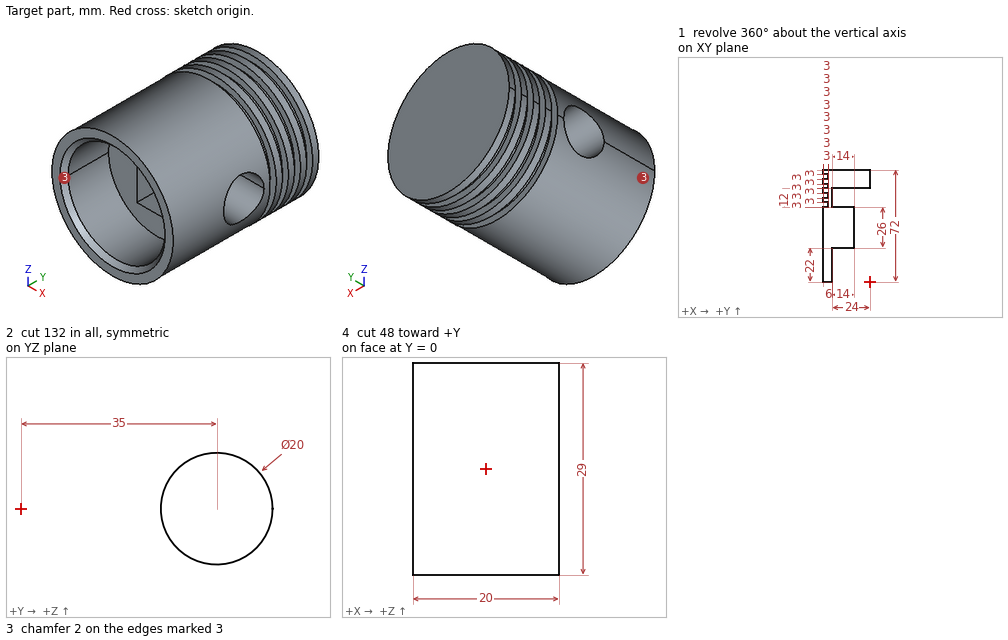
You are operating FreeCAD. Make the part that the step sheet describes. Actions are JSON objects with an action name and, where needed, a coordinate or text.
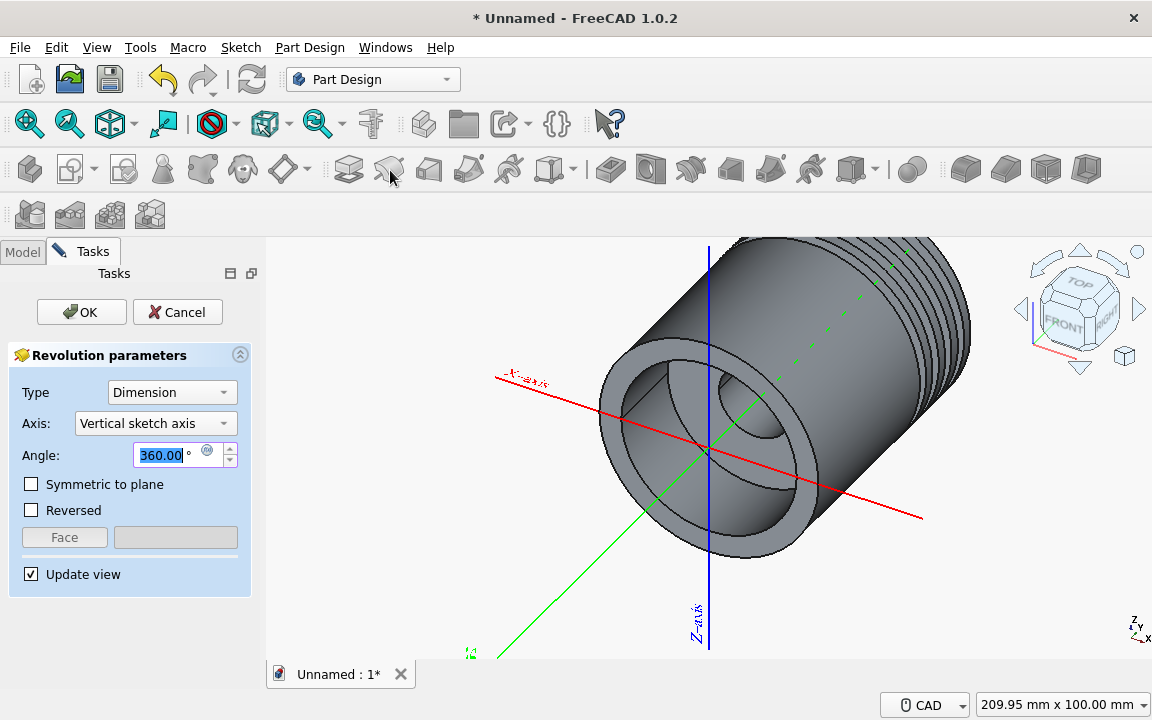
{"action": "left_click", "coordinate": [82, 312]}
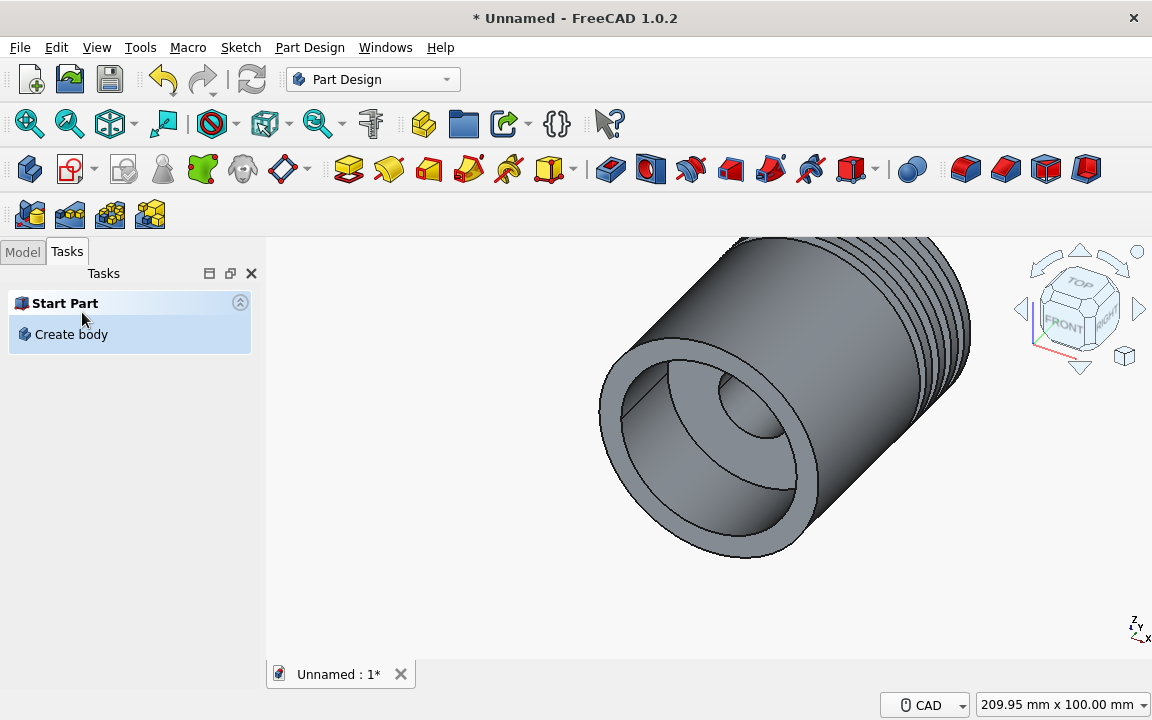
{"action": "left_click", "coordinate": [30, 124]}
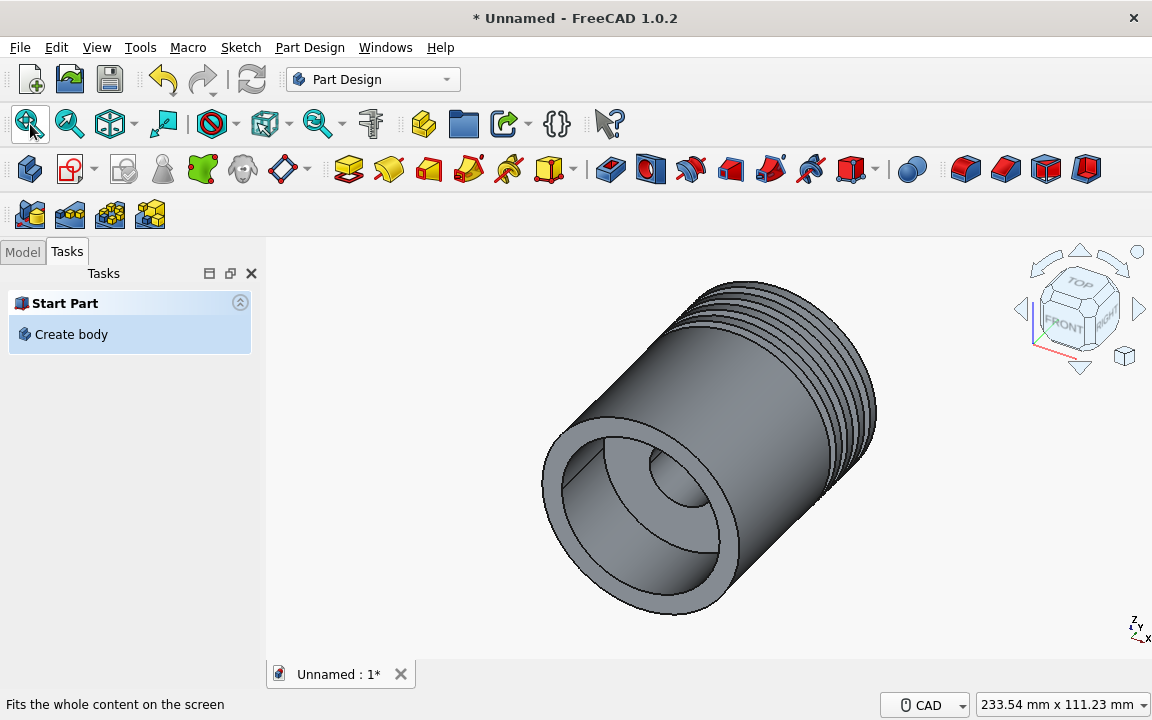
{"action": "left_click", "coordinate": [70, 170]}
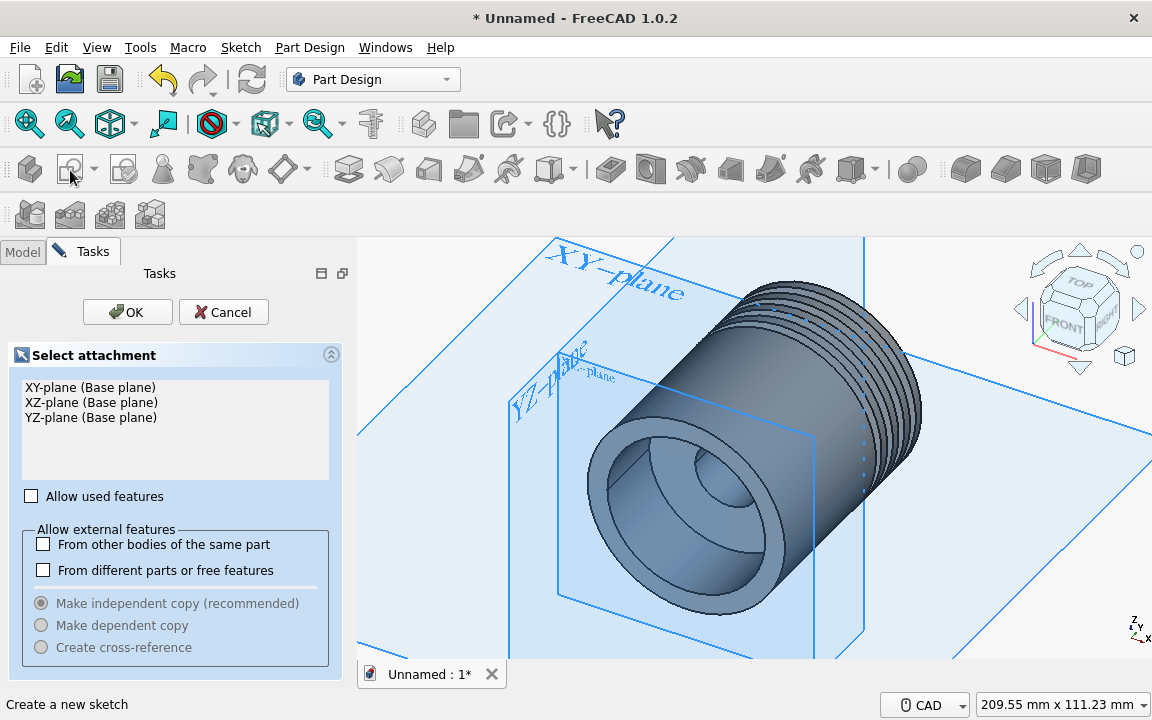
{"action": "left_click", "coordinate": [82, 418]}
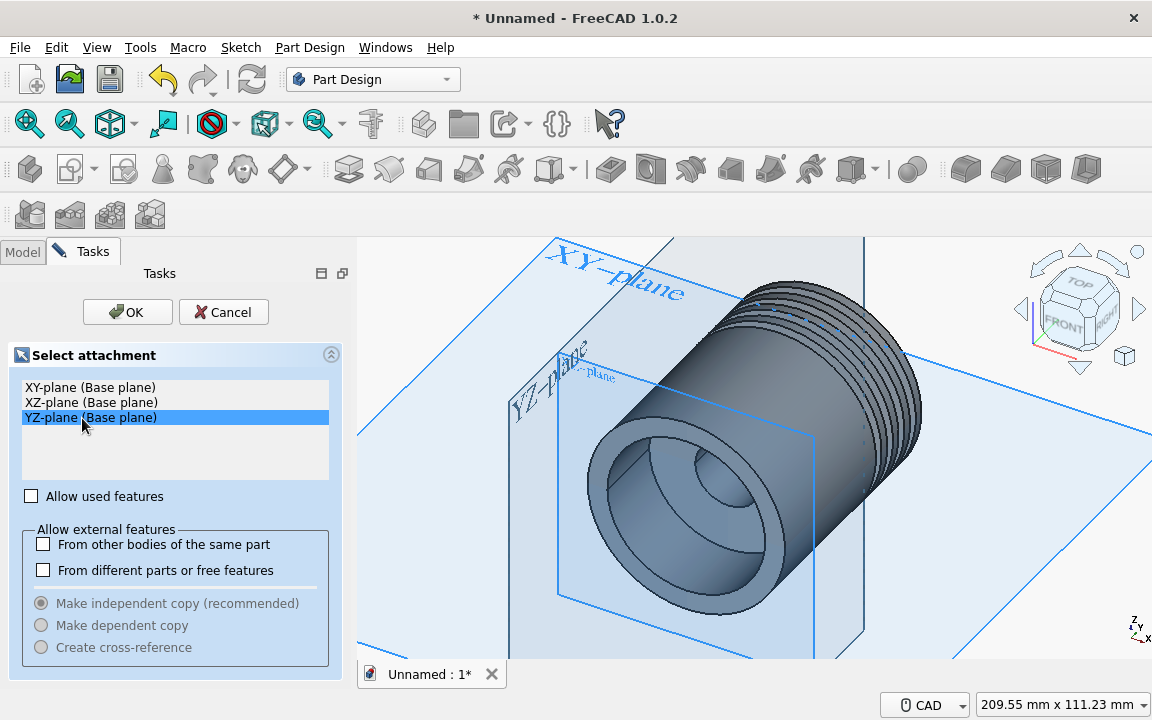
{"action": "left_click", "coordinate": [128, 312]}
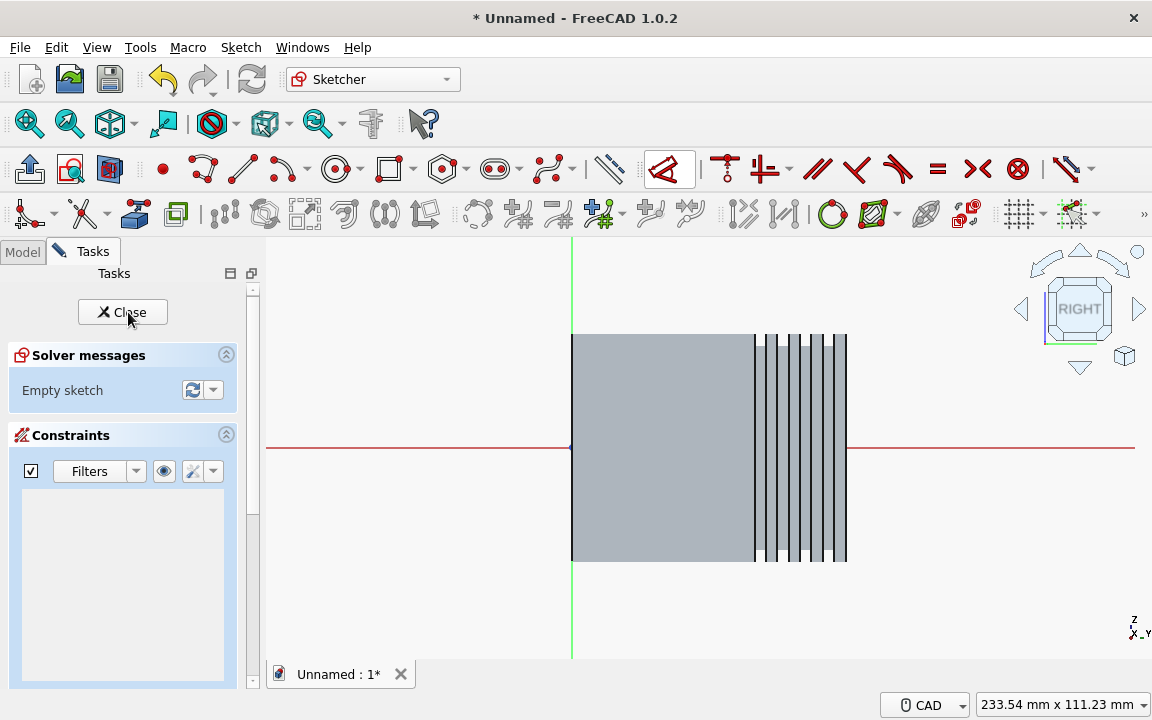
{"action": "left_click", "coordinate": [110, 170]}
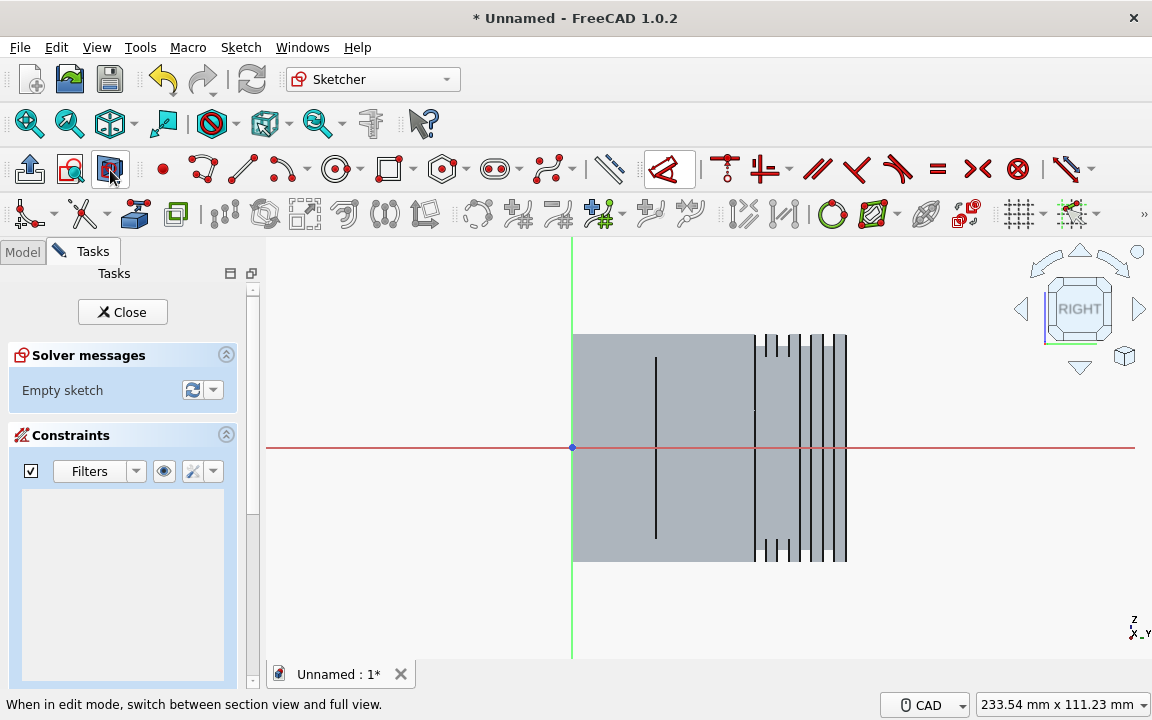
{"action": "scroll", "coordinate": [668, 448], "scroll_direction": "up", "scroll_amount": 5}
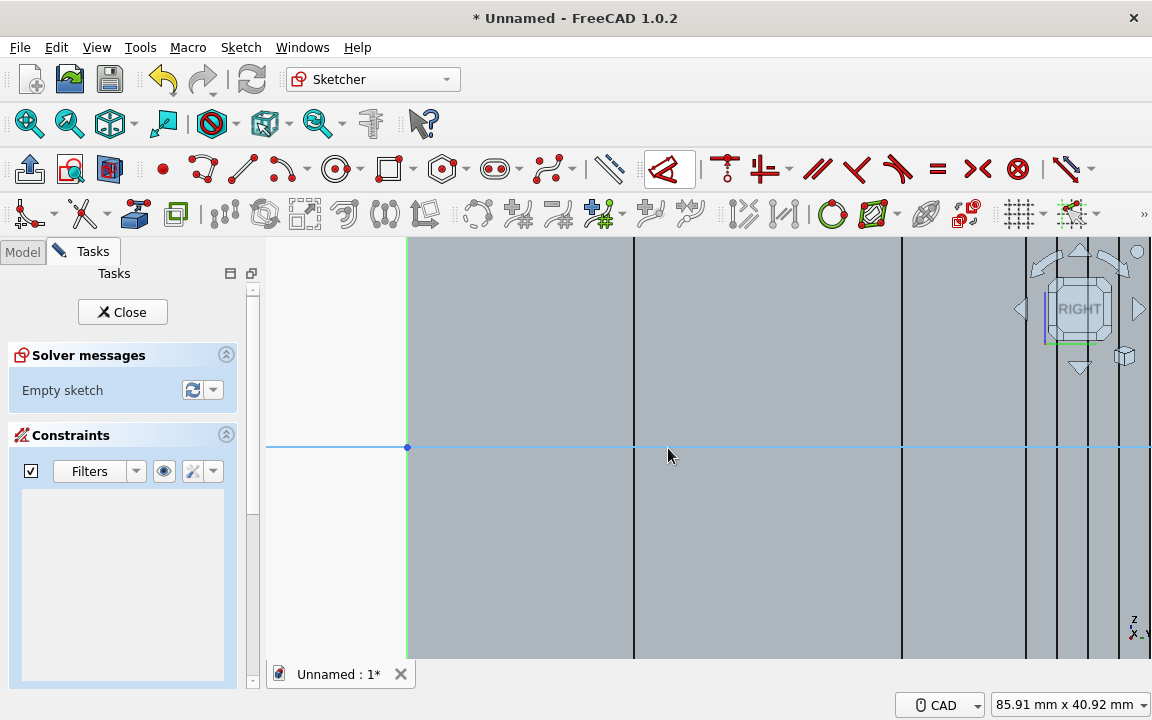
{"action": "left_click", "coordinate": [336, 170]}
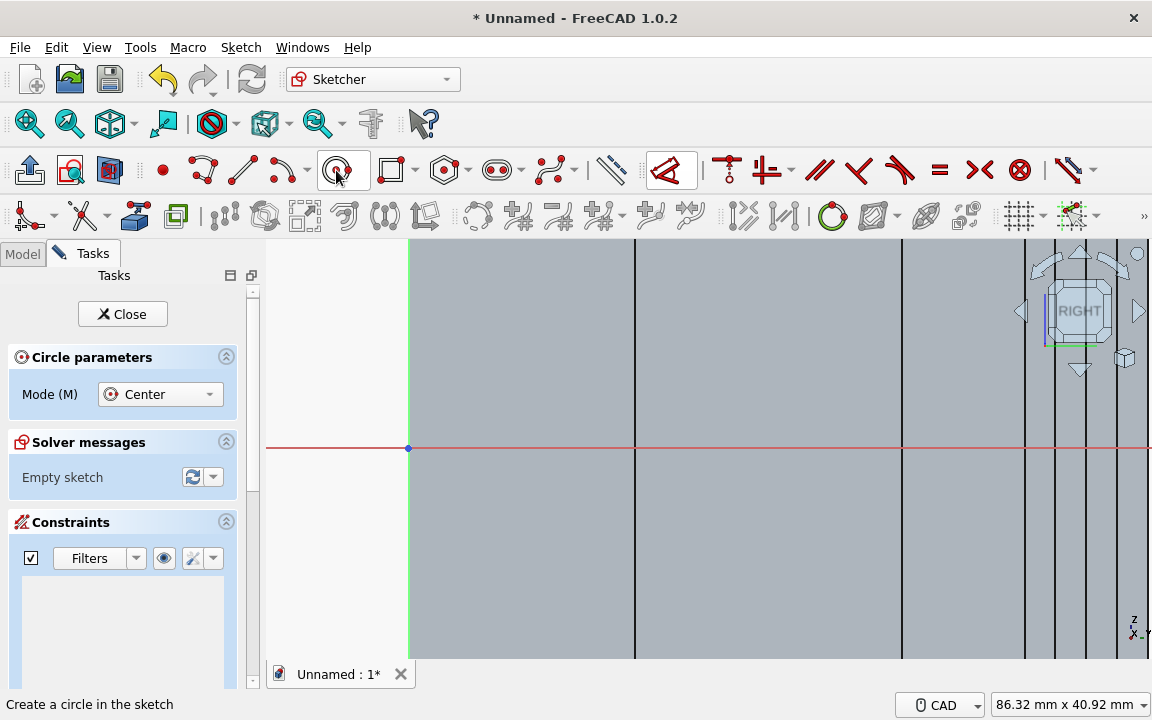
{"action": "left_click", "coordinate": [768, 448]}
{"action": "mouse_move", "coordinate": [841, 376]}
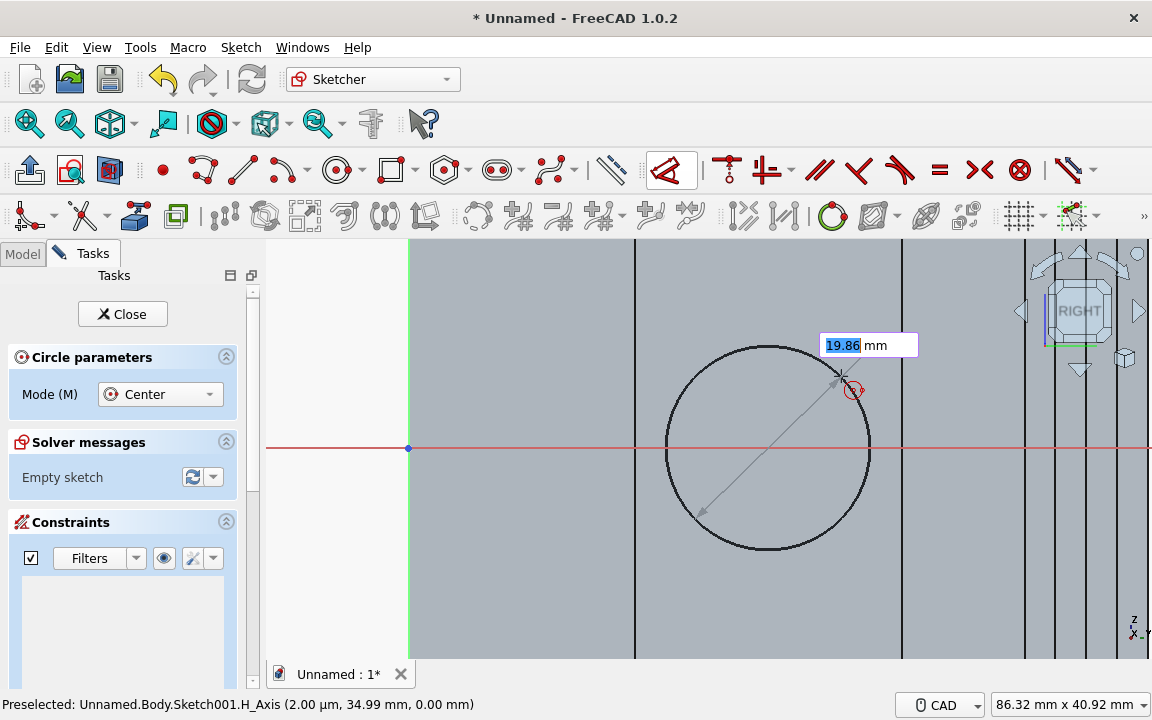
{"action": "type", "text": "20"}
{"action": "key", "text": "Return"}
{"action": "key", "text": "Escape"}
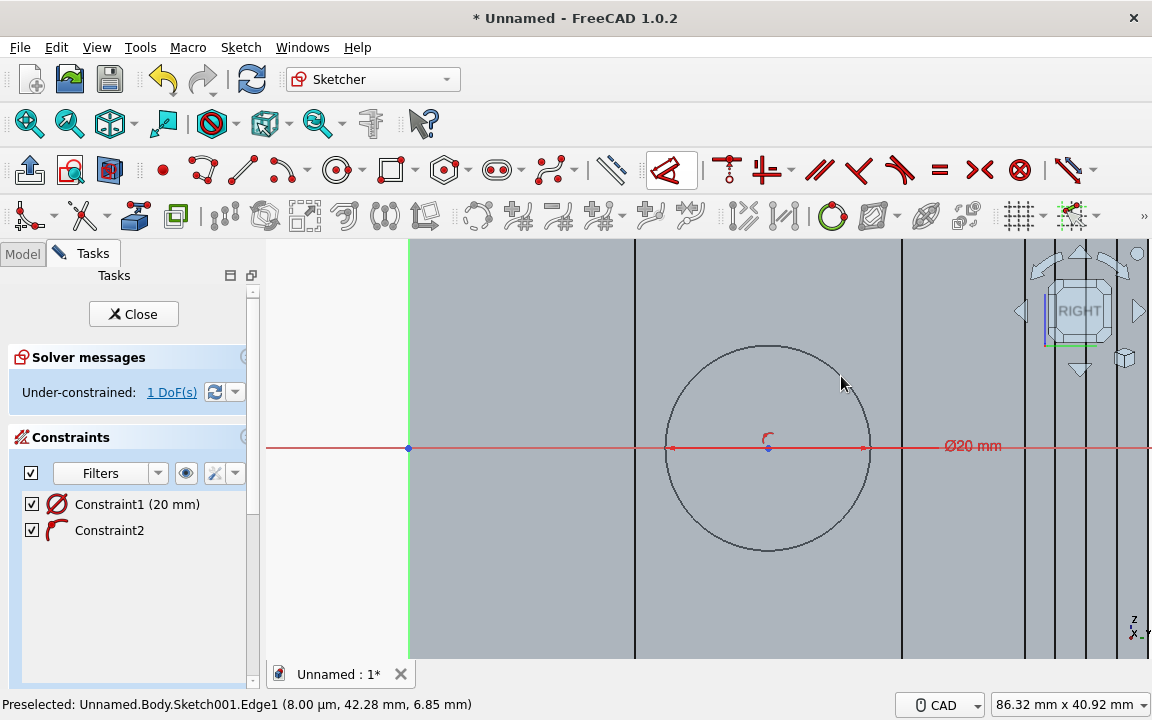
{"action": "left_click", "coordinate": [768, 448]}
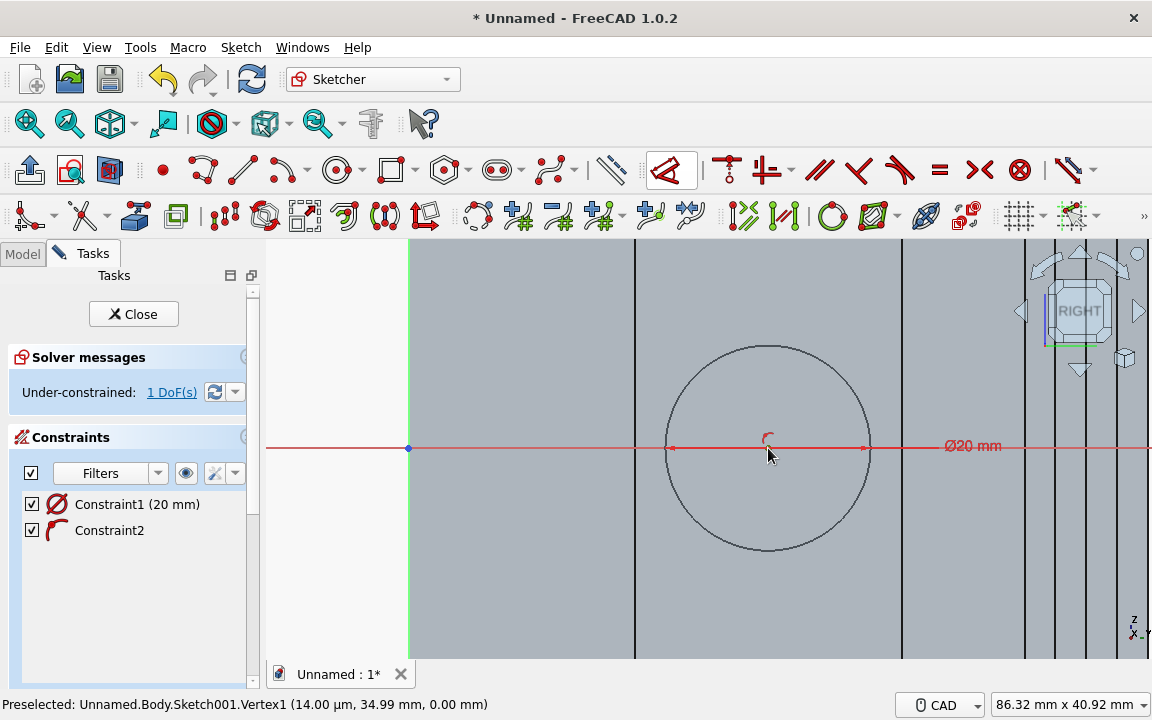
{"action": "key", "text": "l"}